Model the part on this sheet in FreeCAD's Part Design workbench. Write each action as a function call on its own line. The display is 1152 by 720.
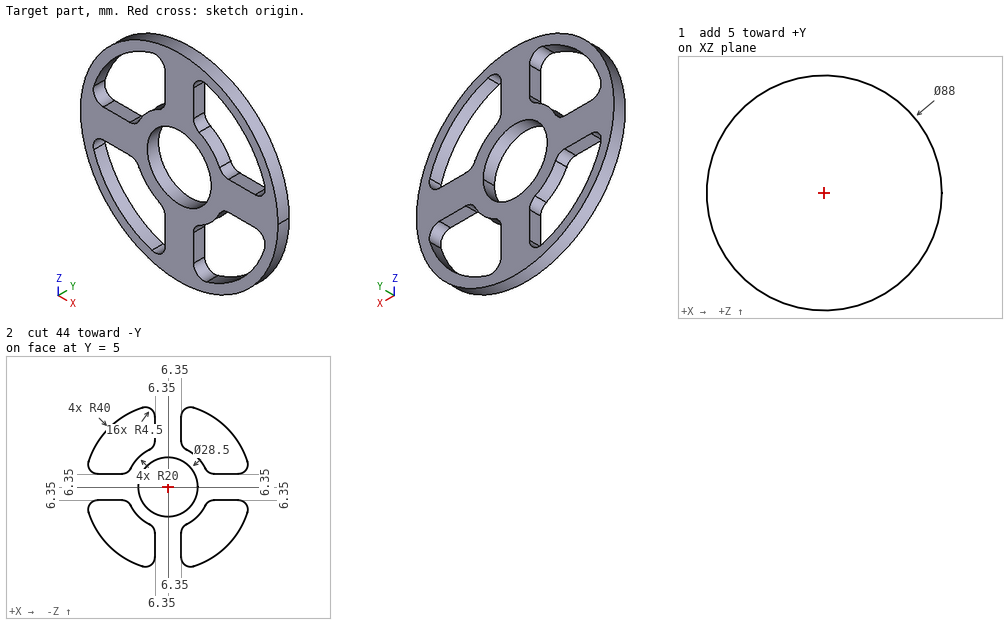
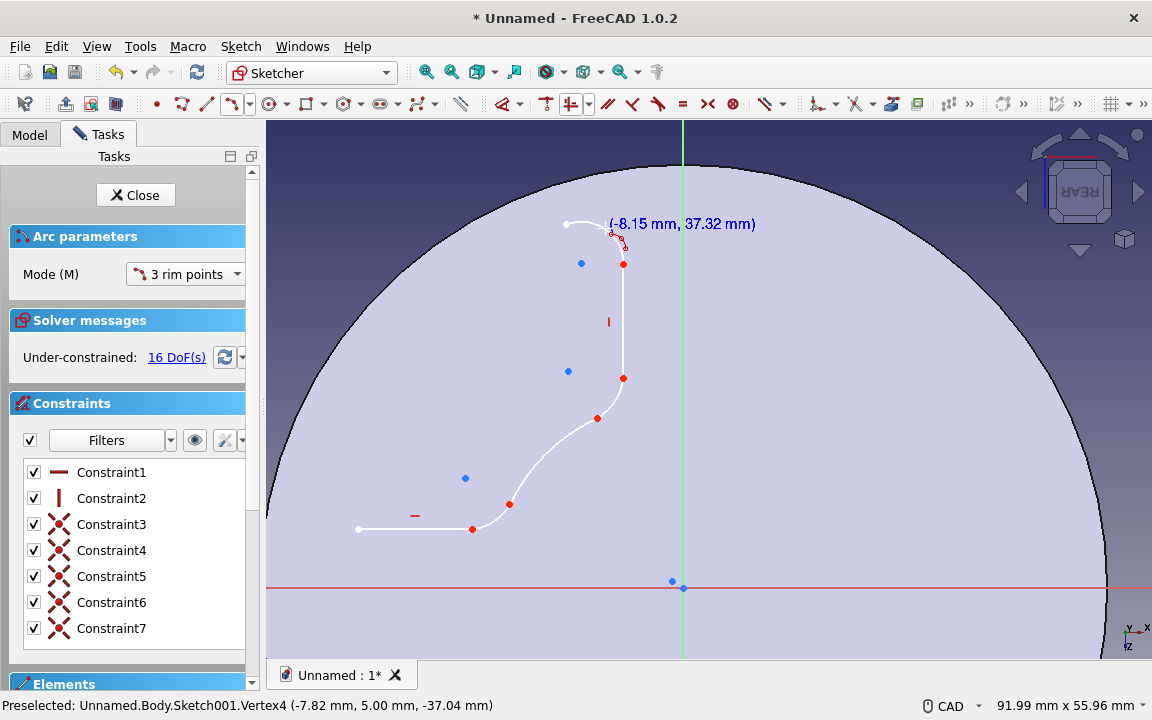
click(567, 225)
click(317, 471)
click(411, 316)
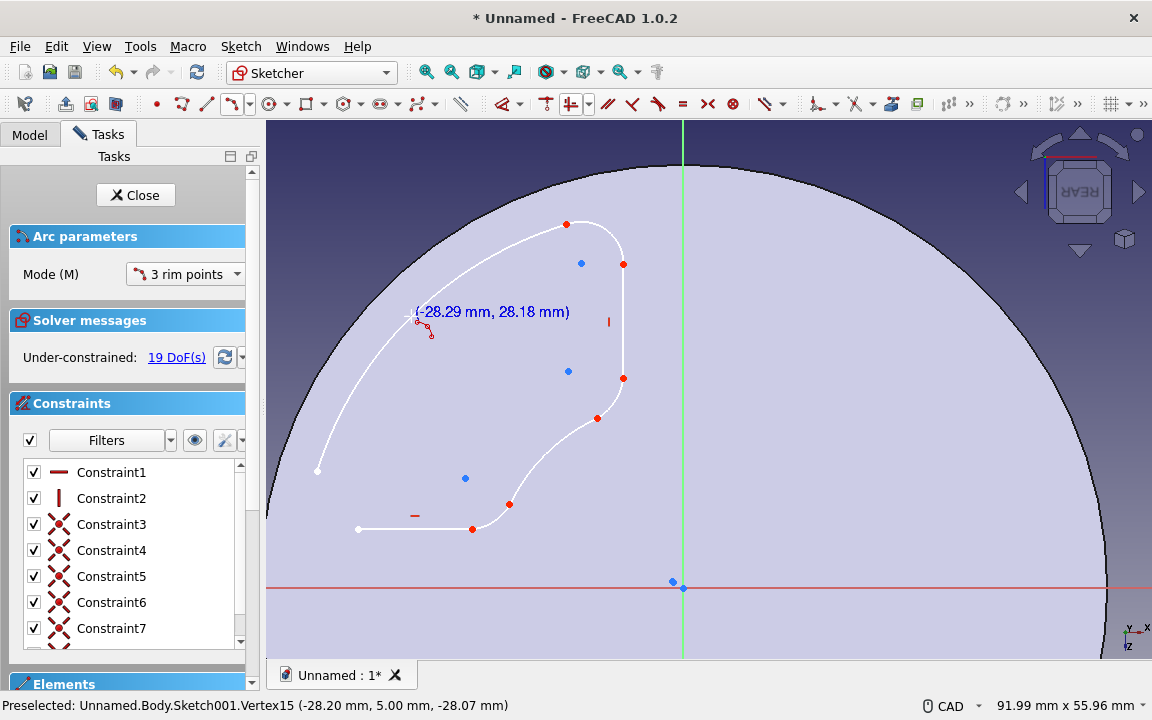
click(317, 472)
click(359, 529)
click(323, 509)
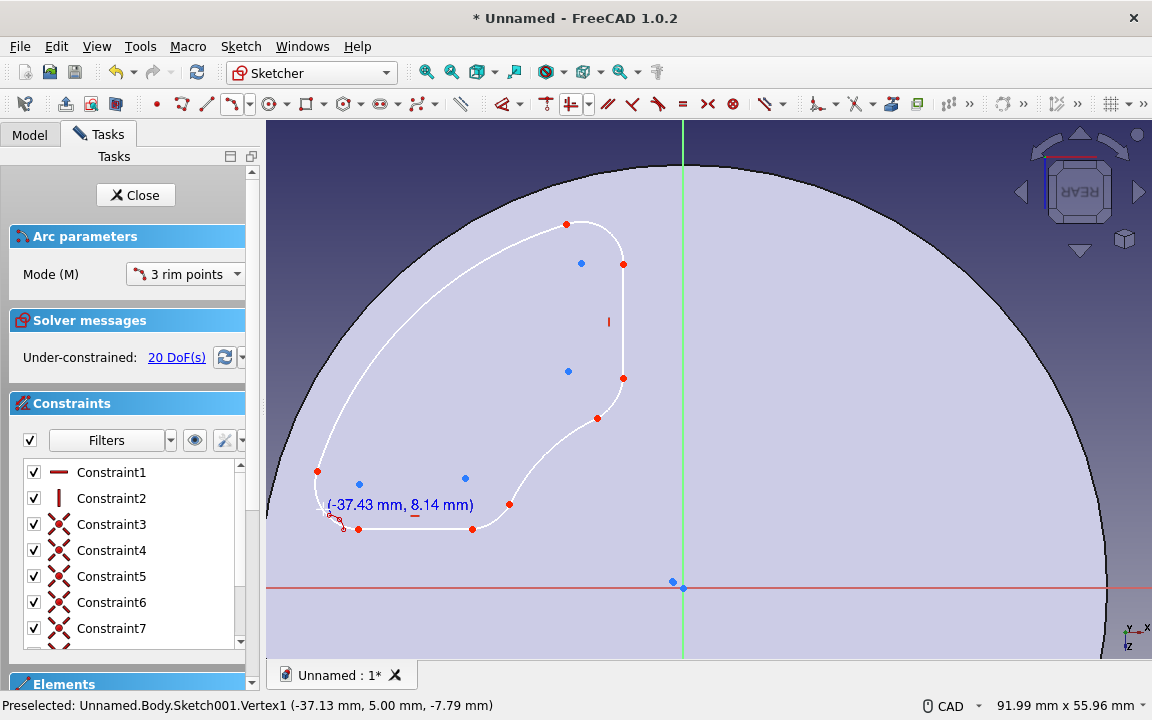
key(g)
key(l)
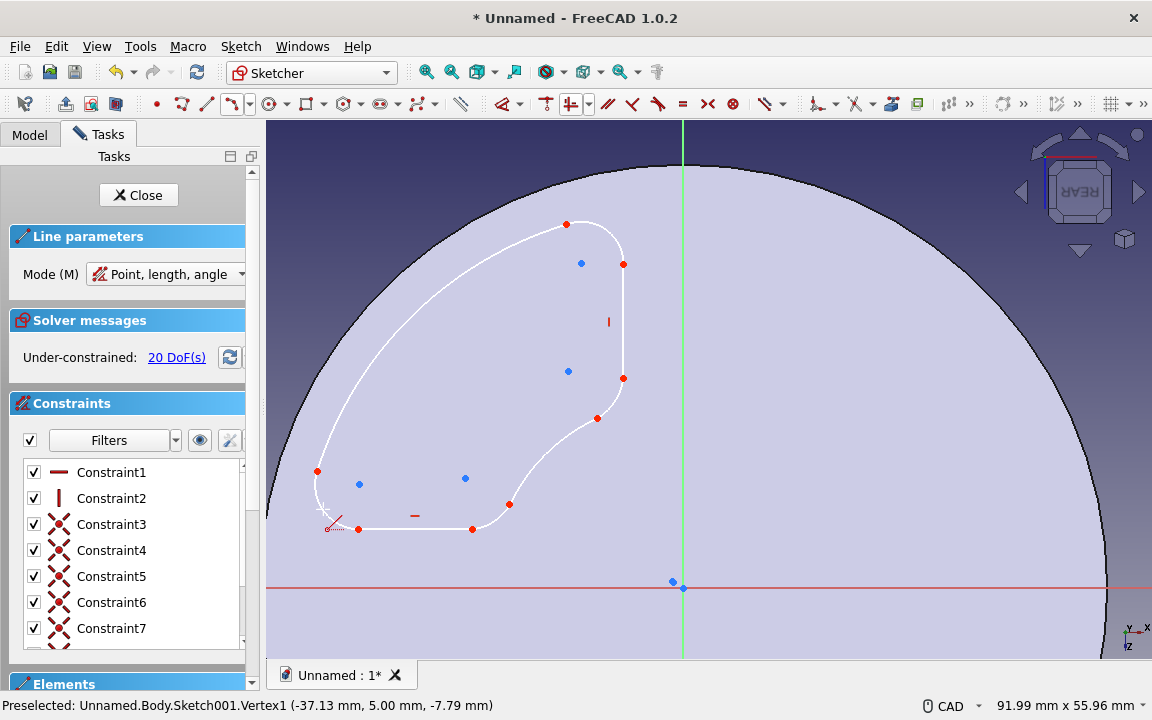
click(895, 527)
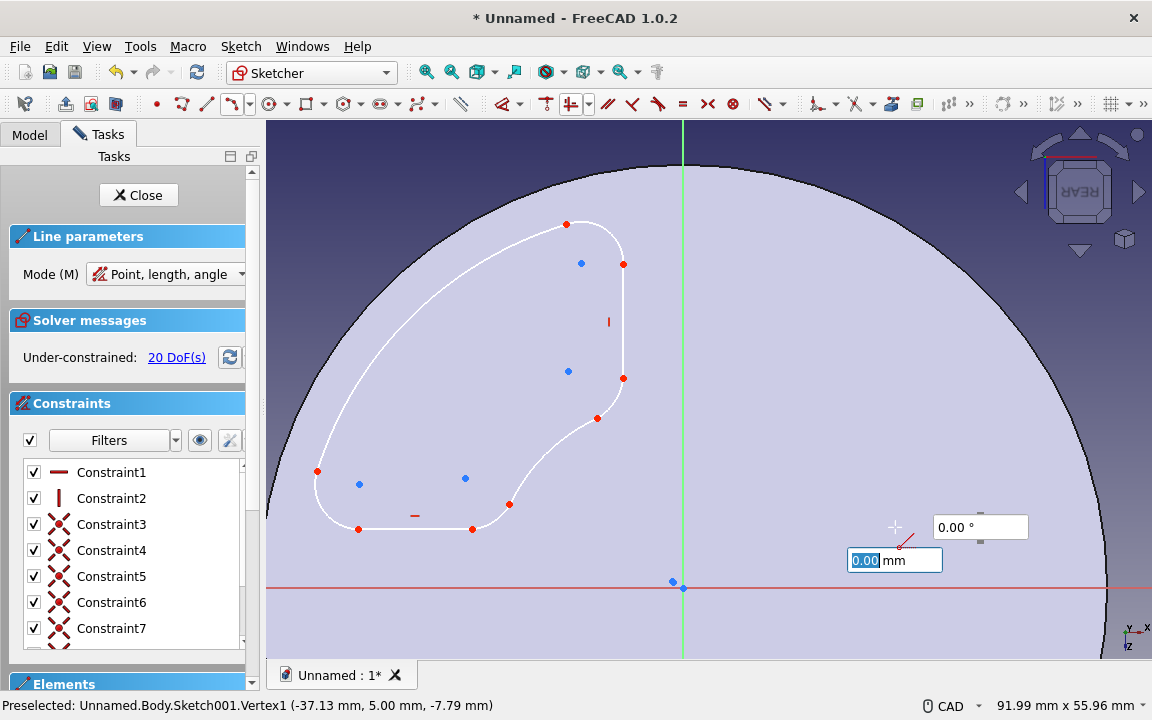
scroll(605, 227, down, 4)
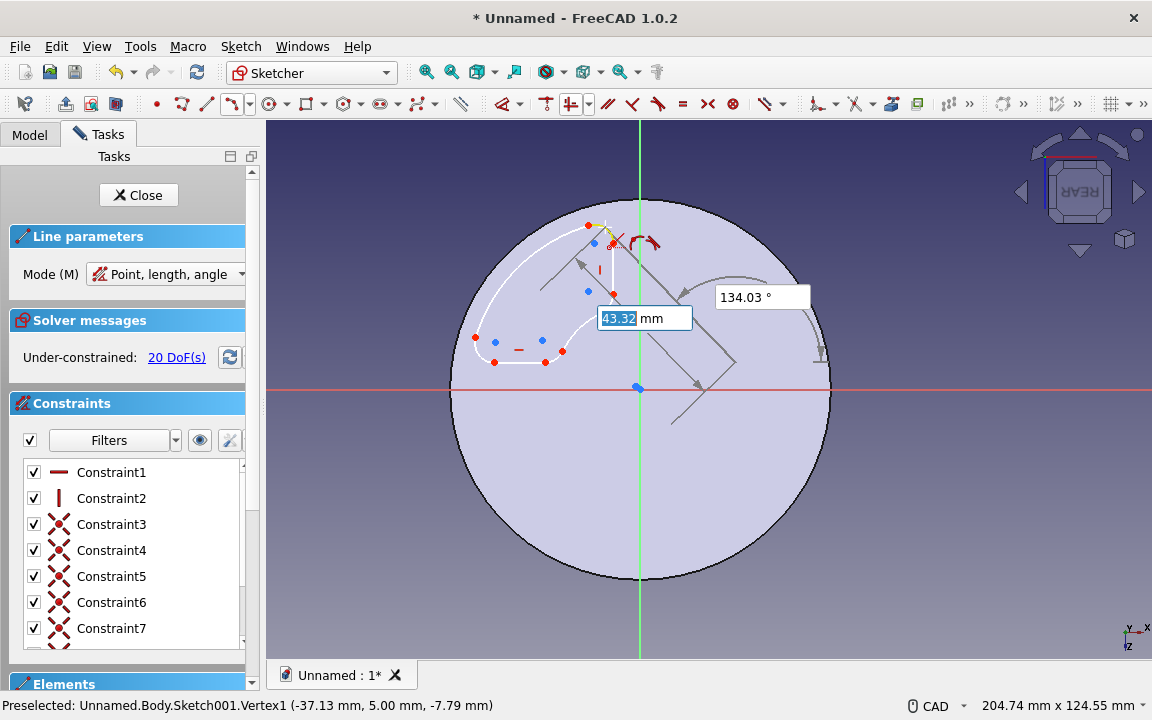
click(787, 362)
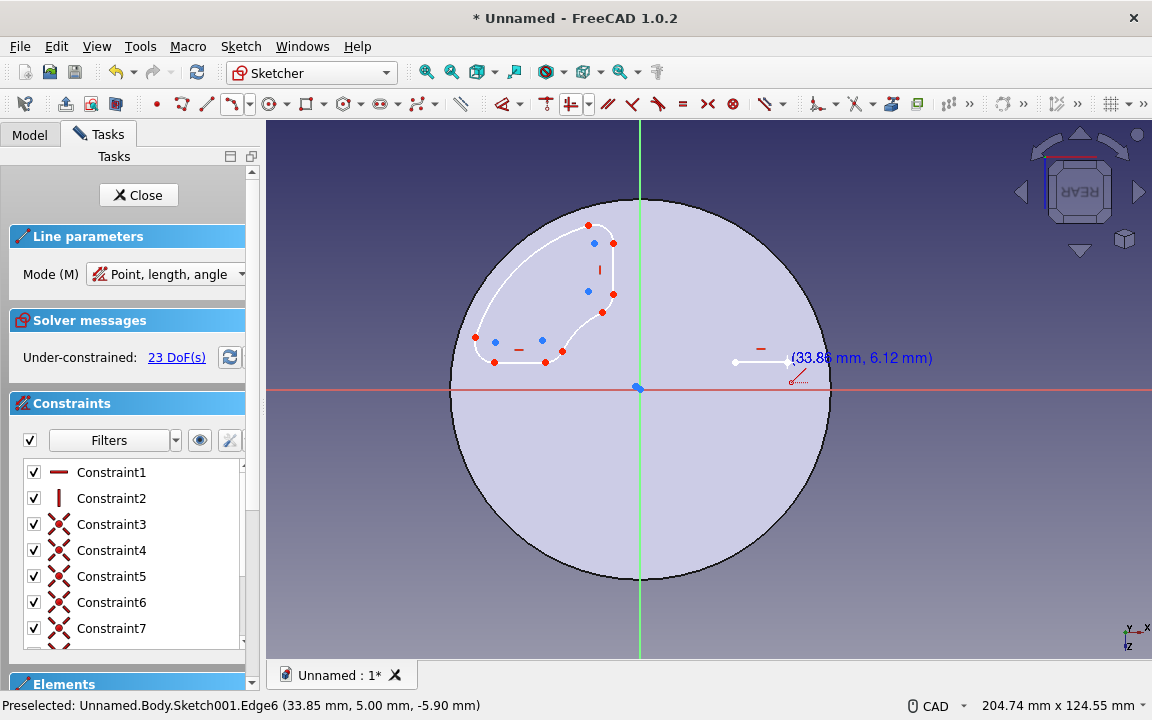
click(668, 243)
click(668, 294)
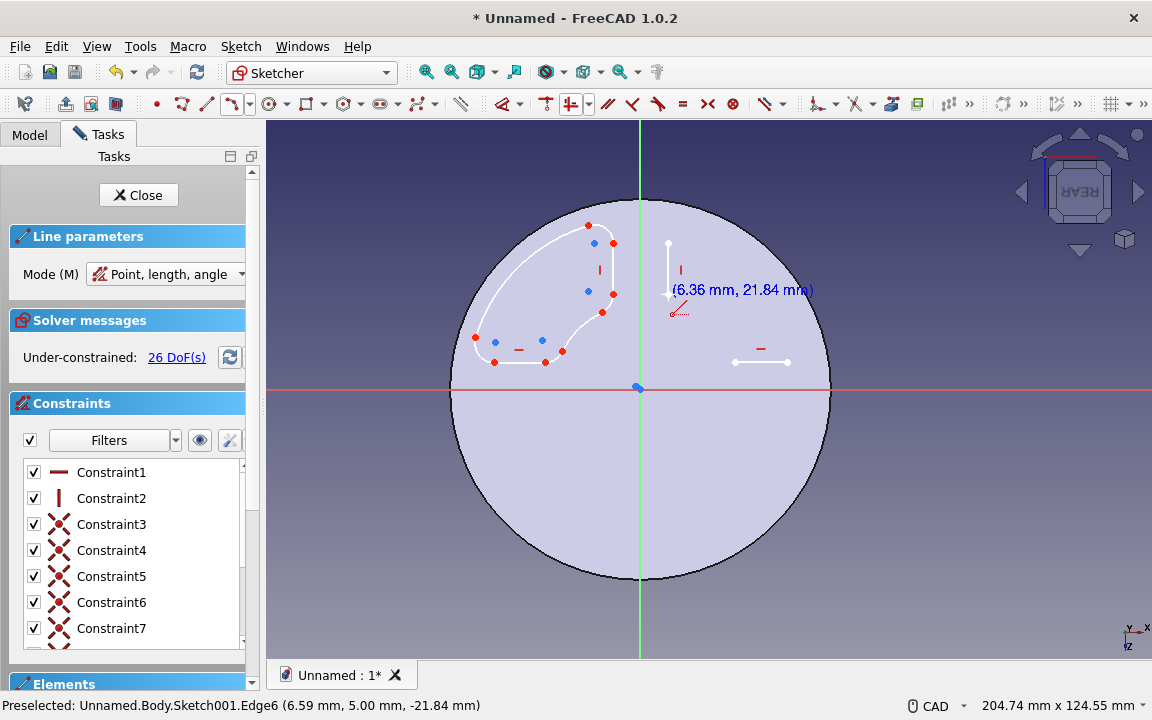
key(g)
key(3)
key(a)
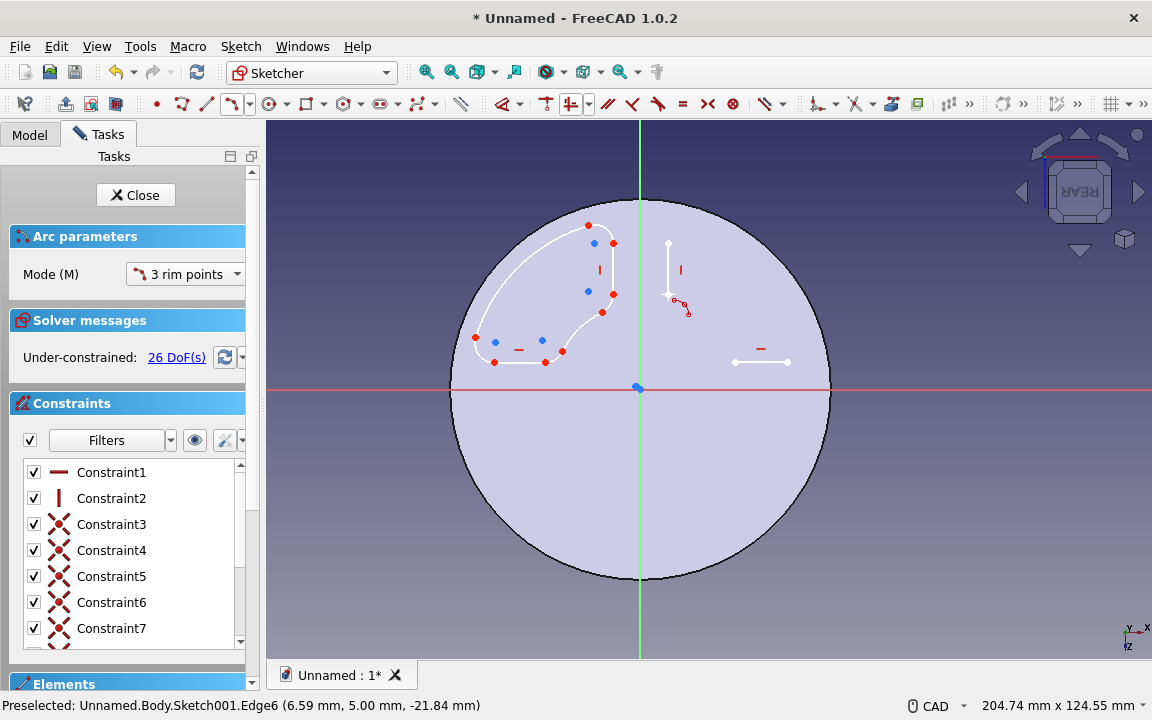
click(787, 362)
click(805, 337)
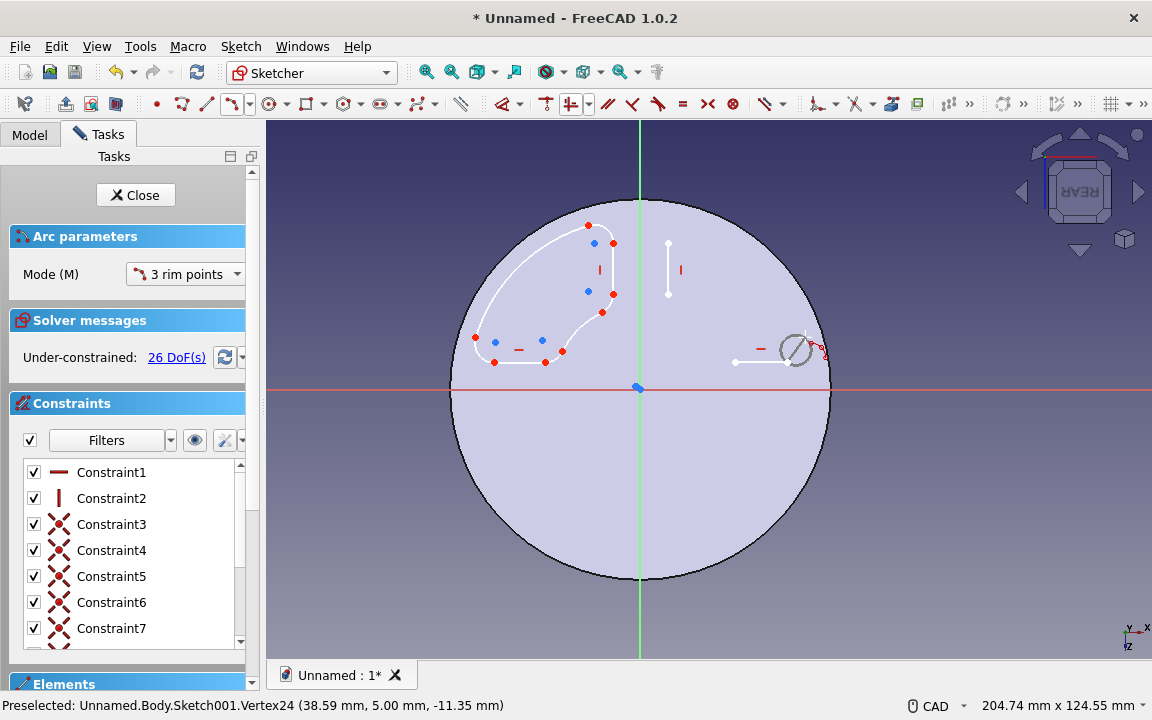
scroll(802, 354, up, 4)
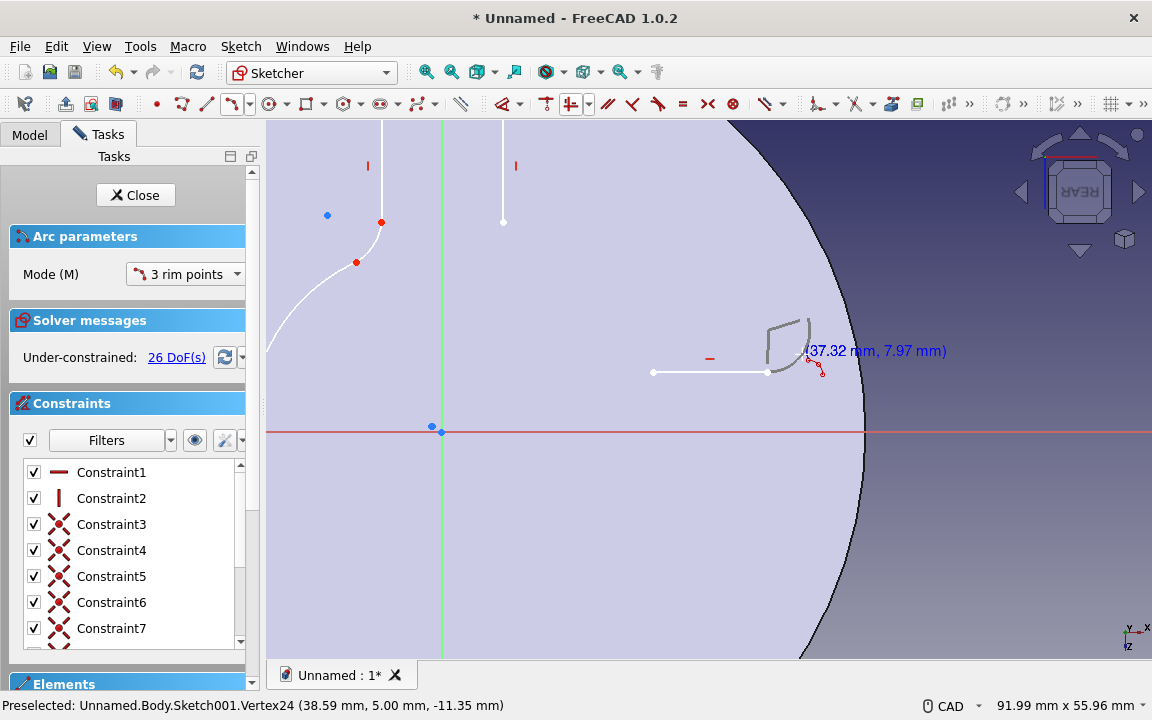
click(802, 354)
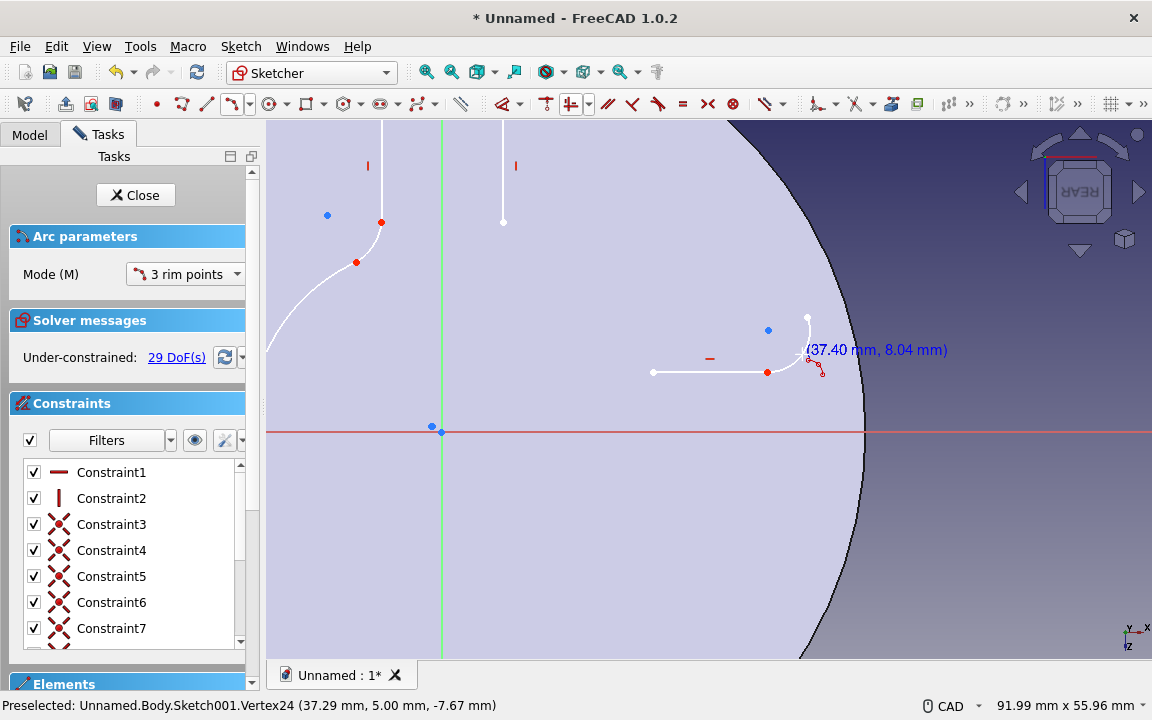
click(808, 318)